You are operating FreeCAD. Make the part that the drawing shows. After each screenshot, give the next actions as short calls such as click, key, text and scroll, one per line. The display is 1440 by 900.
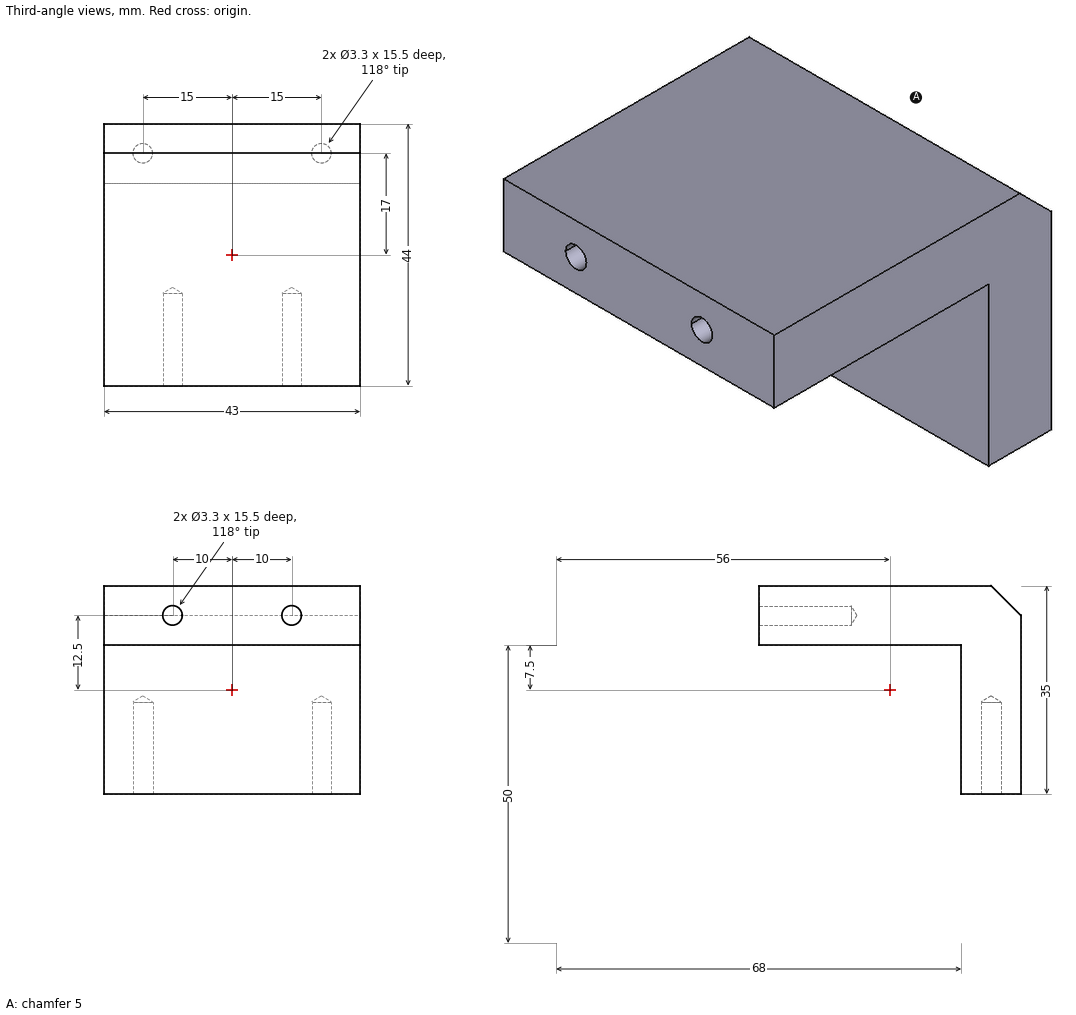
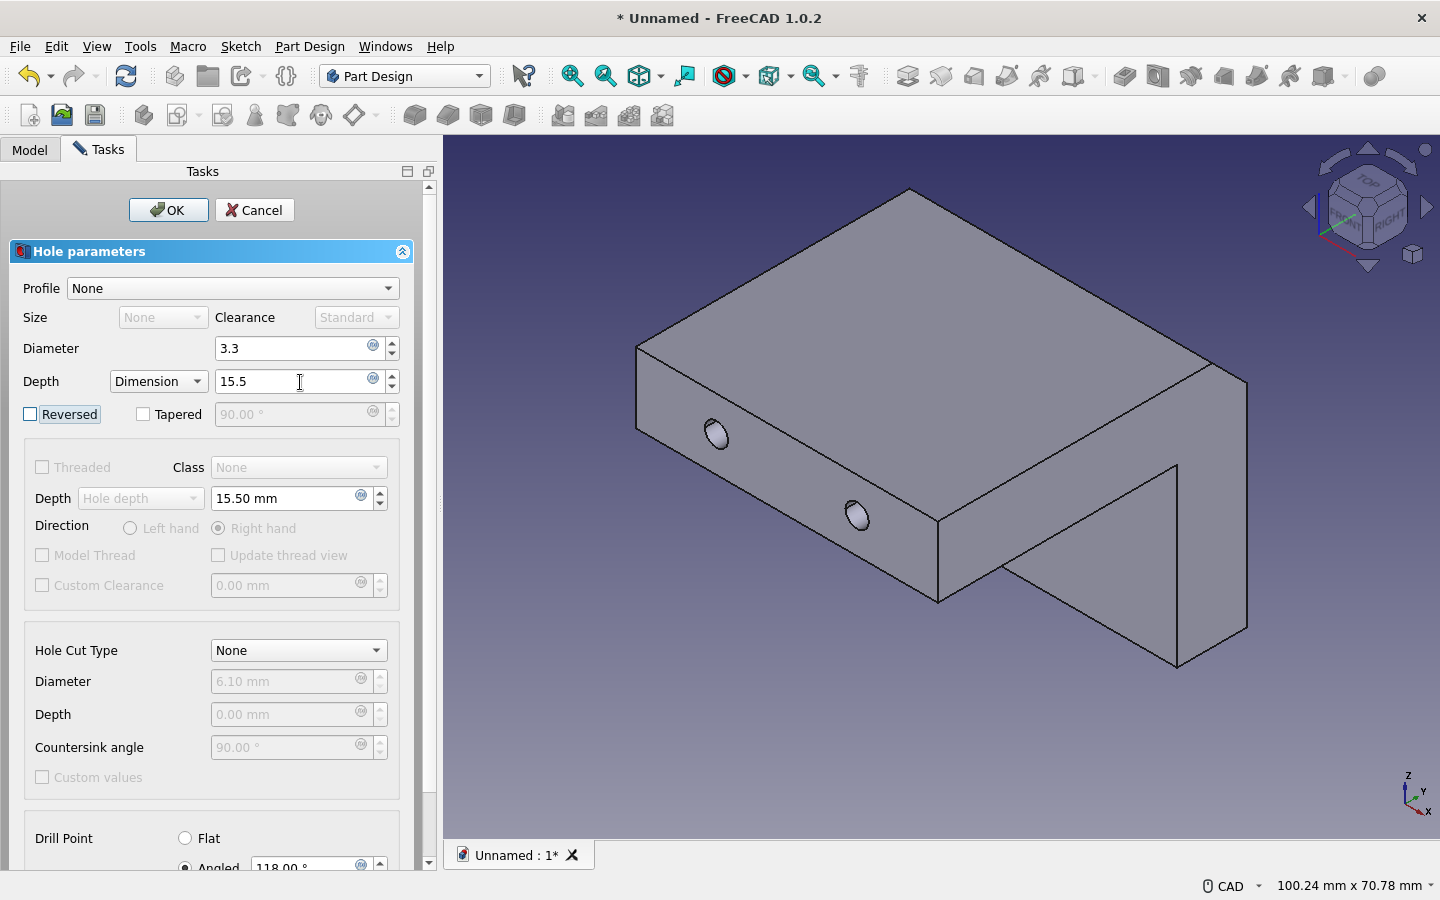
click(169, 210)